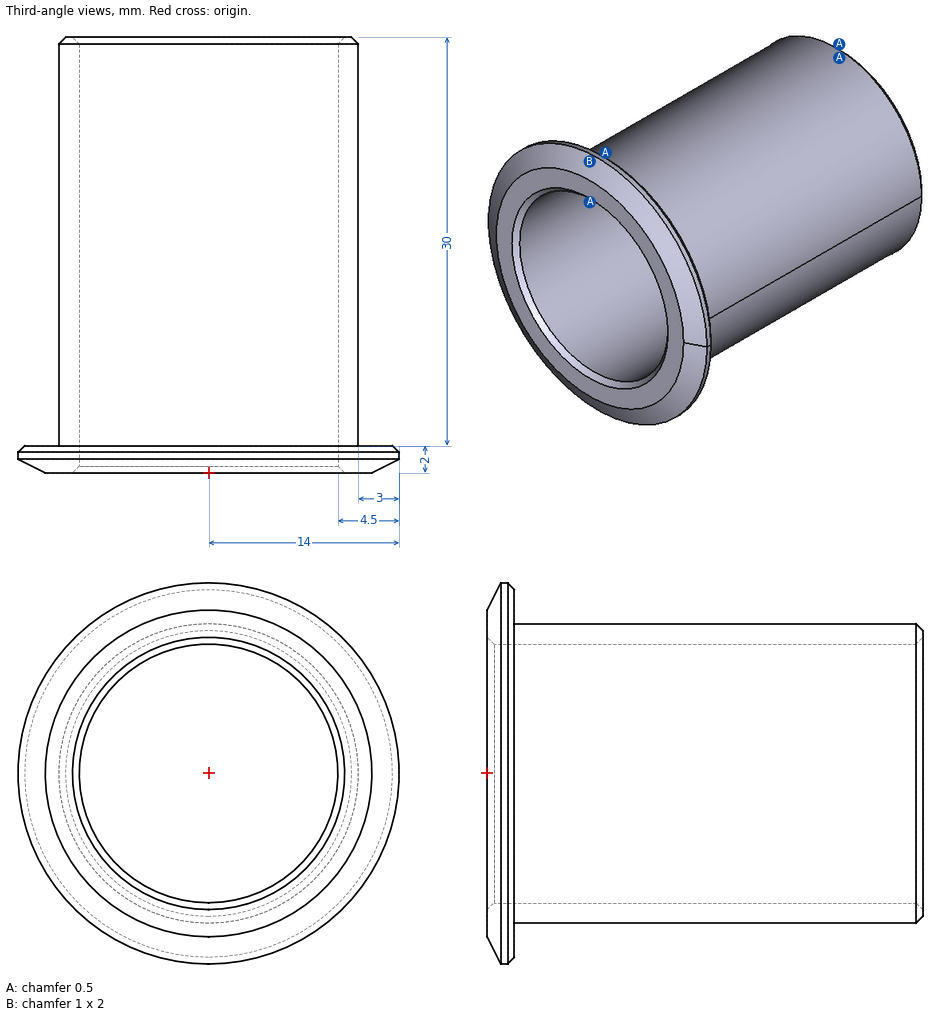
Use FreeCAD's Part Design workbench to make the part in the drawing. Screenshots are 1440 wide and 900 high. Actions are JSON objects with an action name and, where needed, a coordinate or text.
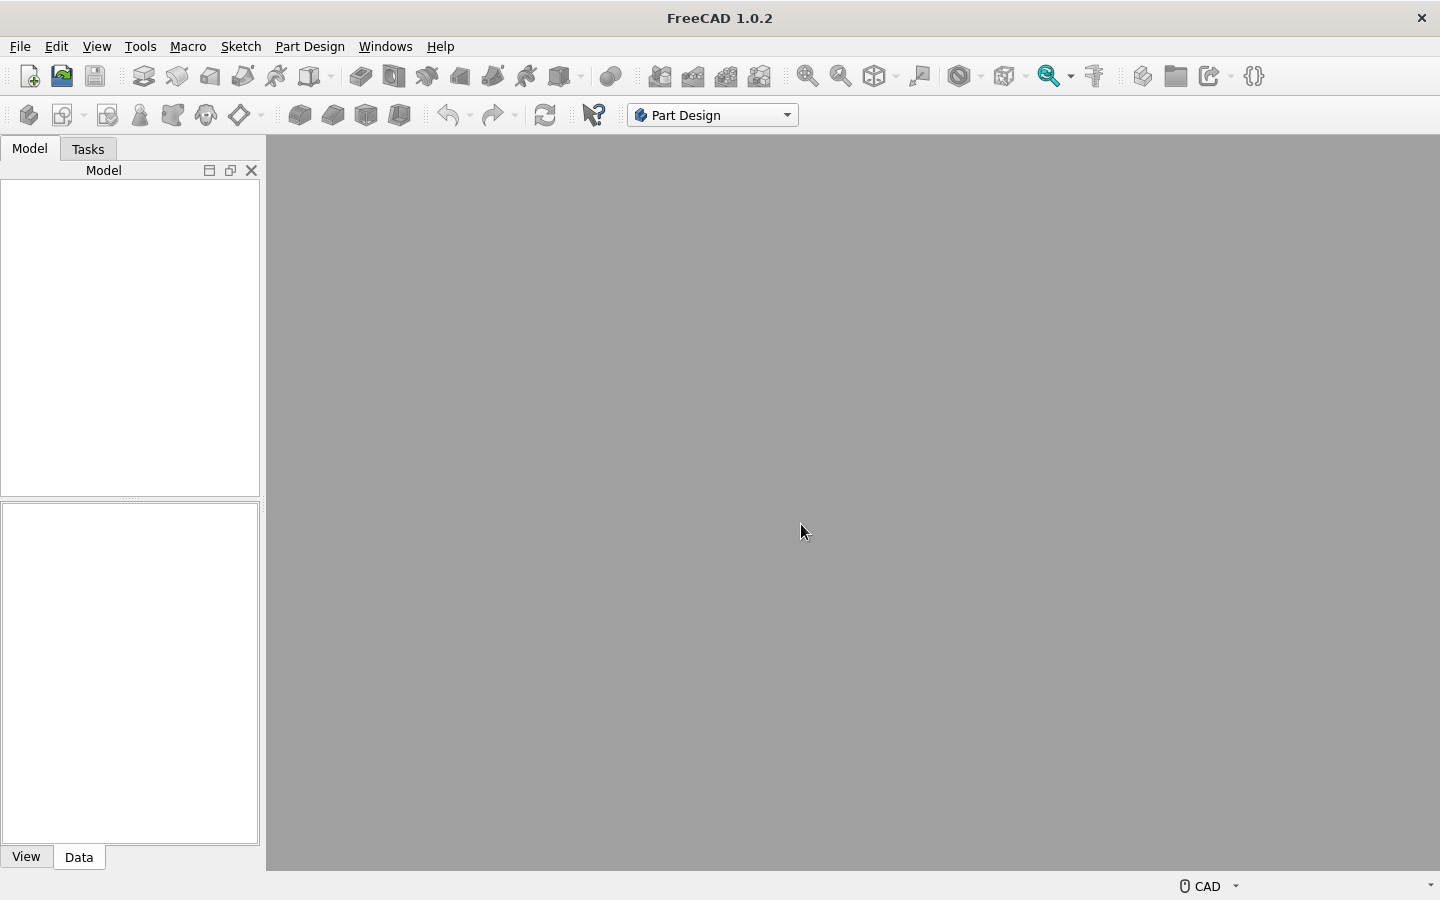
{"action": "key", "text": "ctrl+n"}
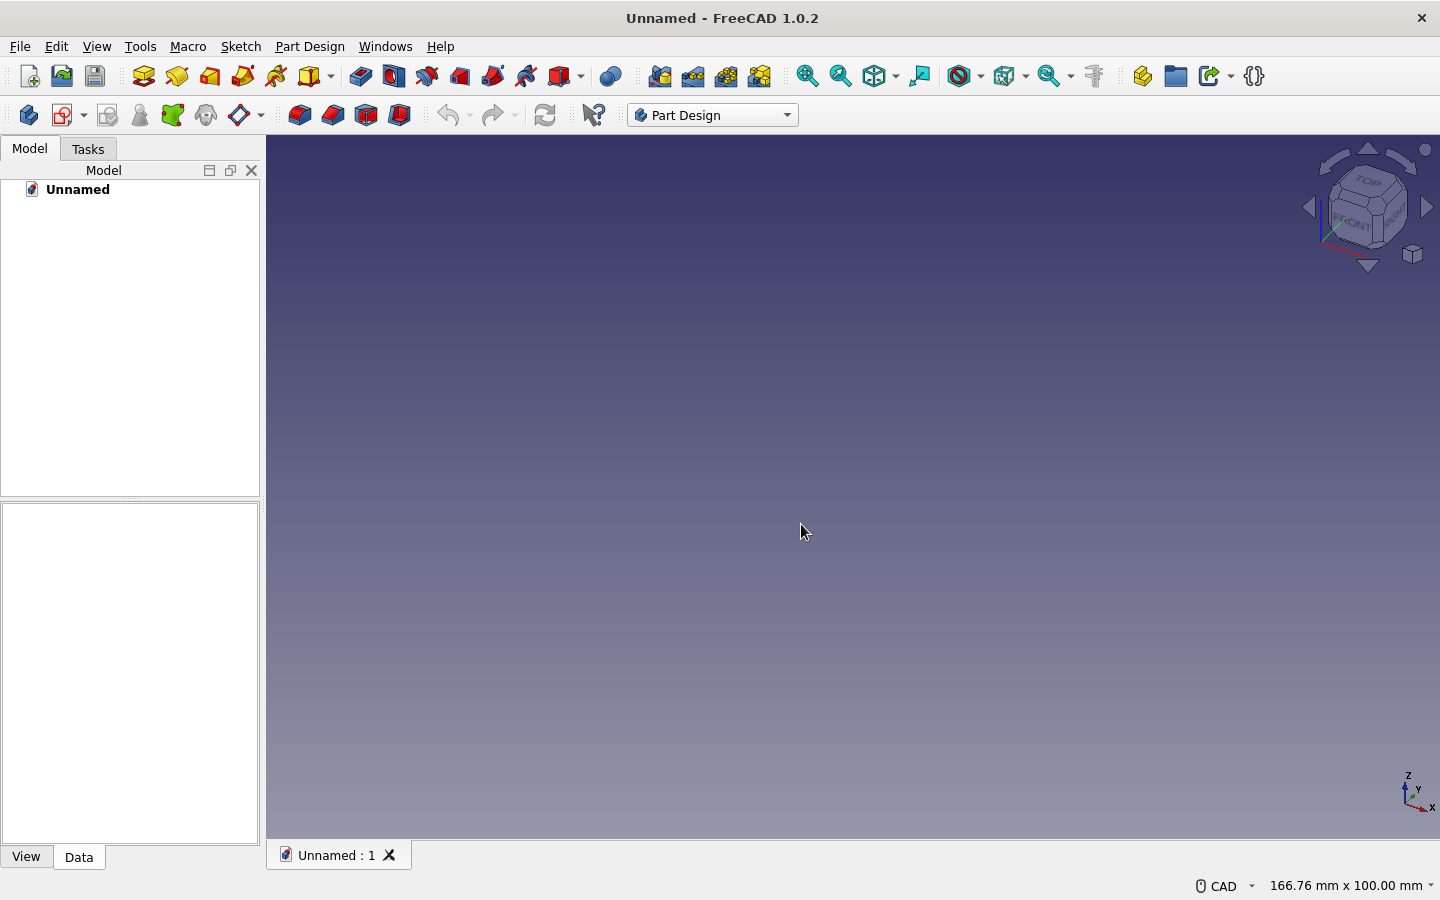
{"action": "left_click", "coordinate": [62, 116]}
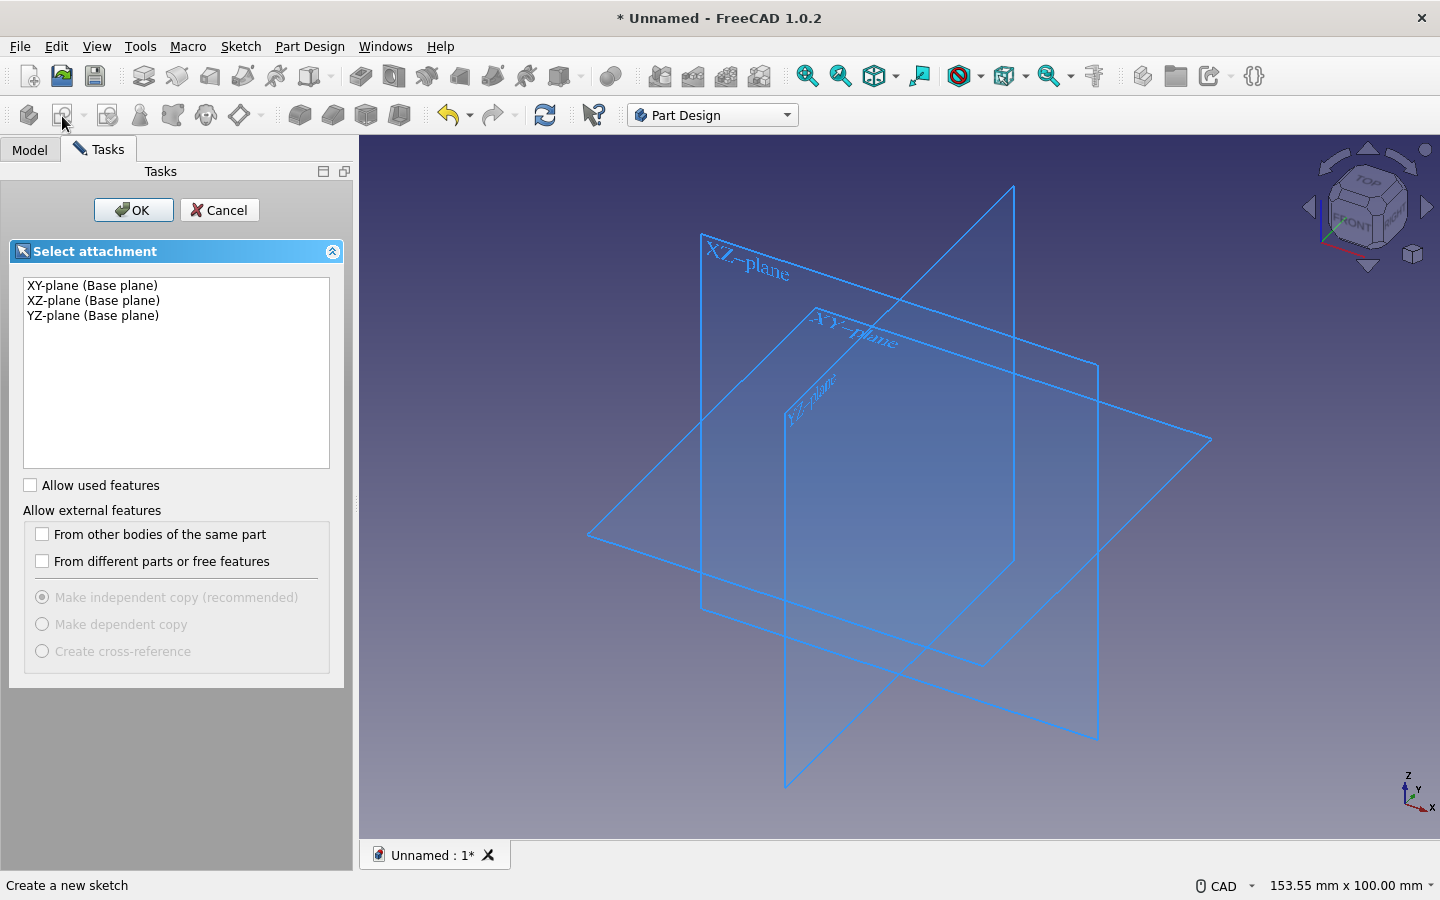
{"action": "left_click", "coordinate": [84, 286]}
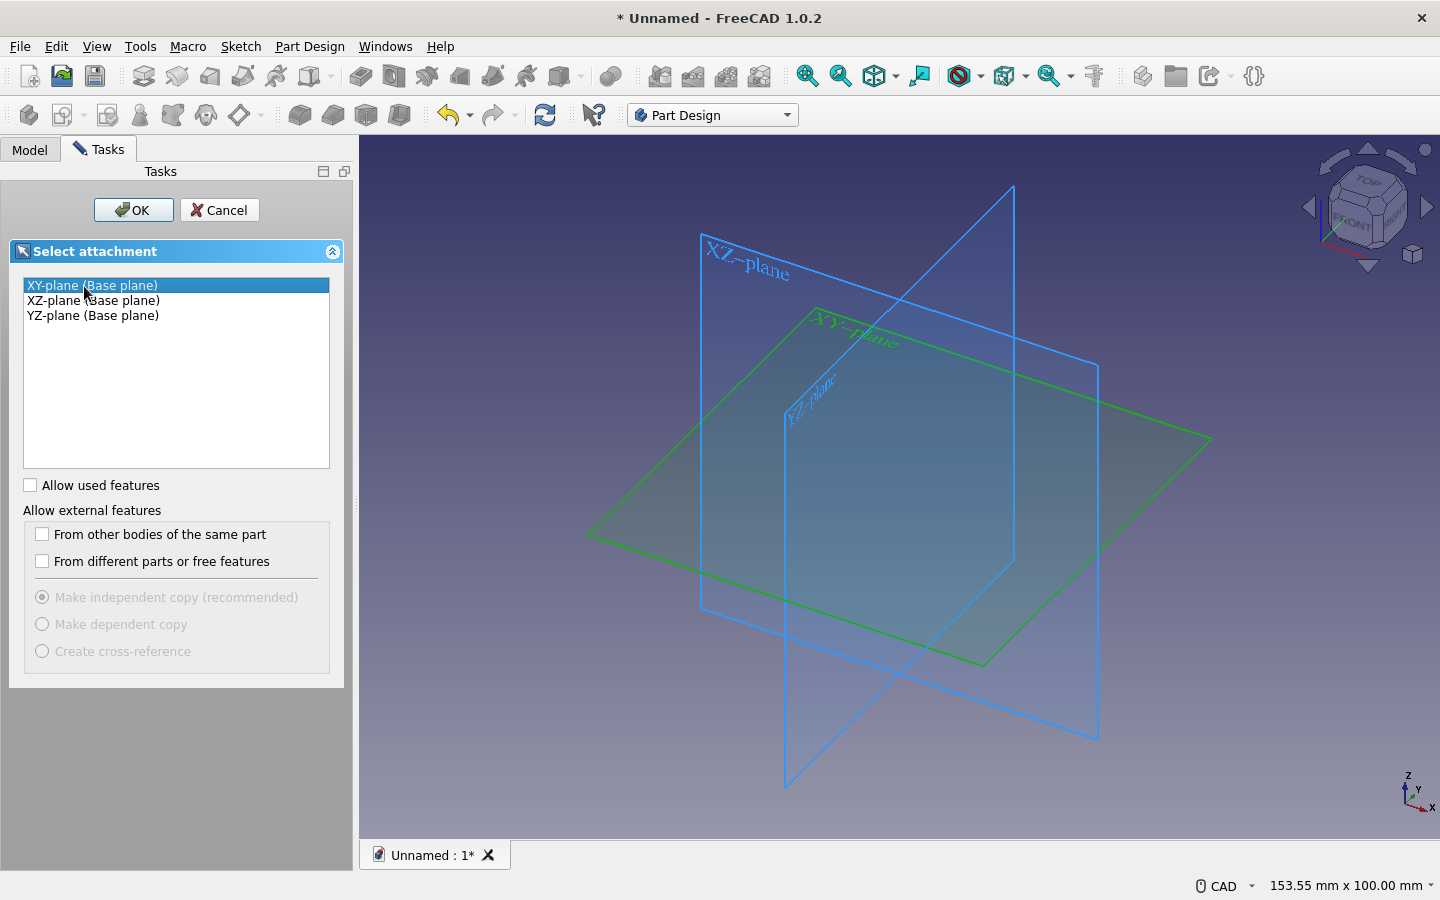
{"action": "left_click", "coordinate": [134, 210]}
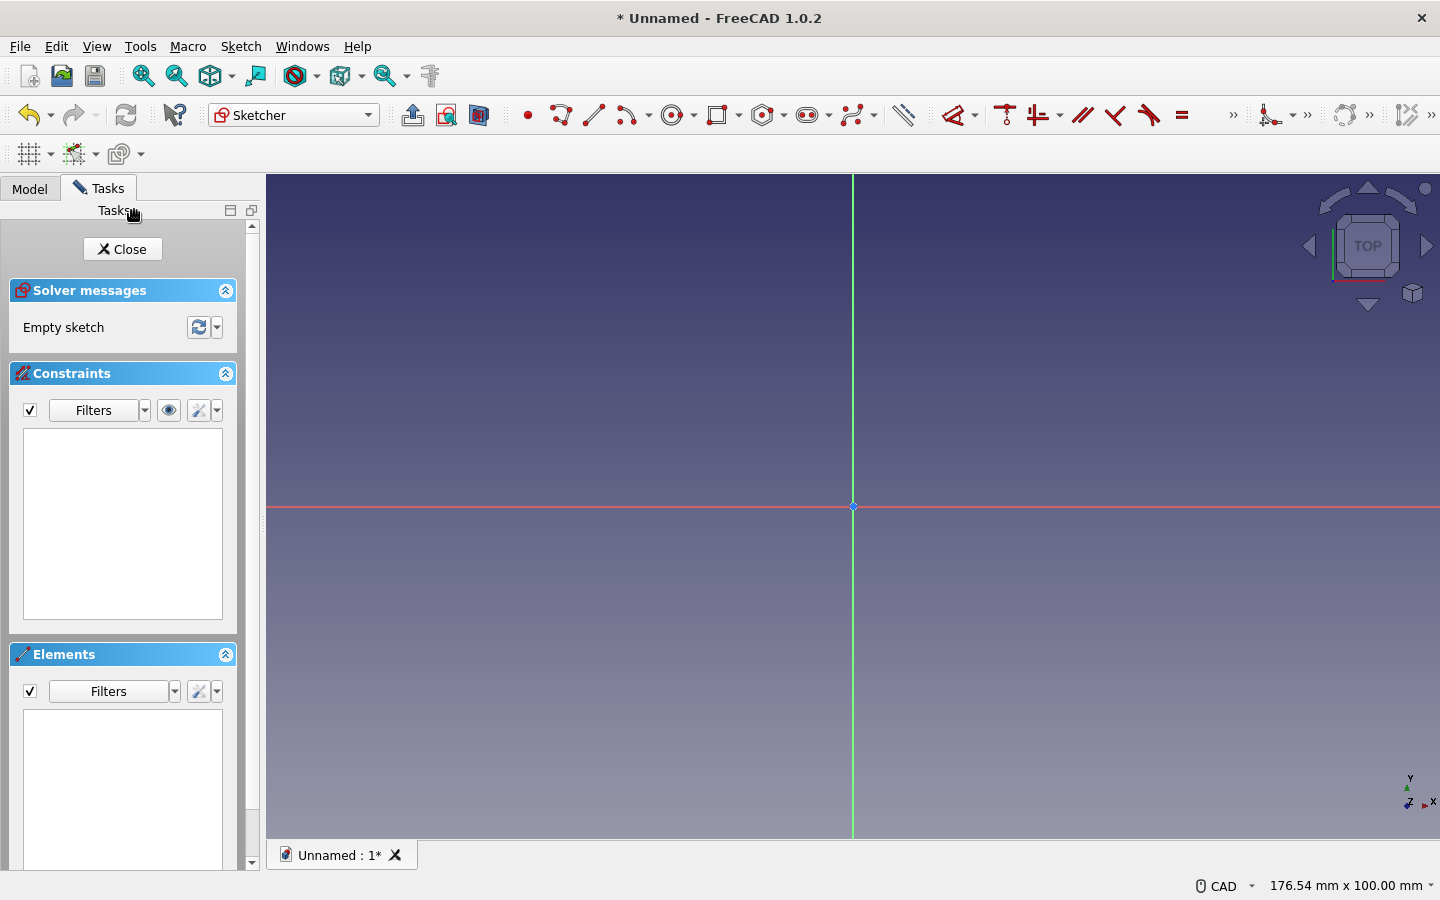
{"action": "scroll", "coordinate": [993, 313], "scroll_direction": "up", "scroll_amount": 4}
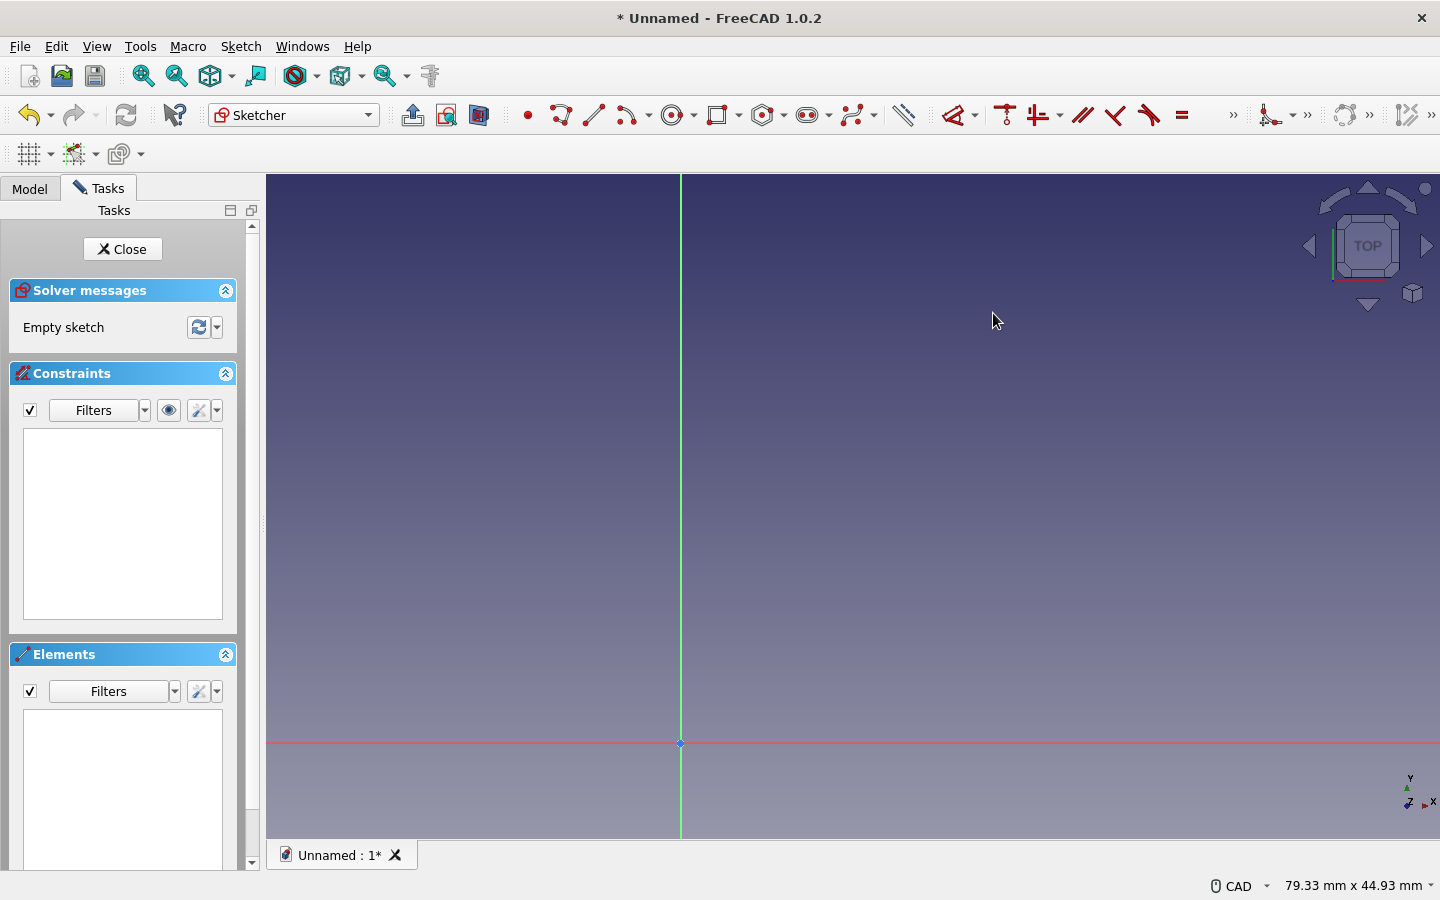
{"action": "left_click", "coordinate": [561, 116]}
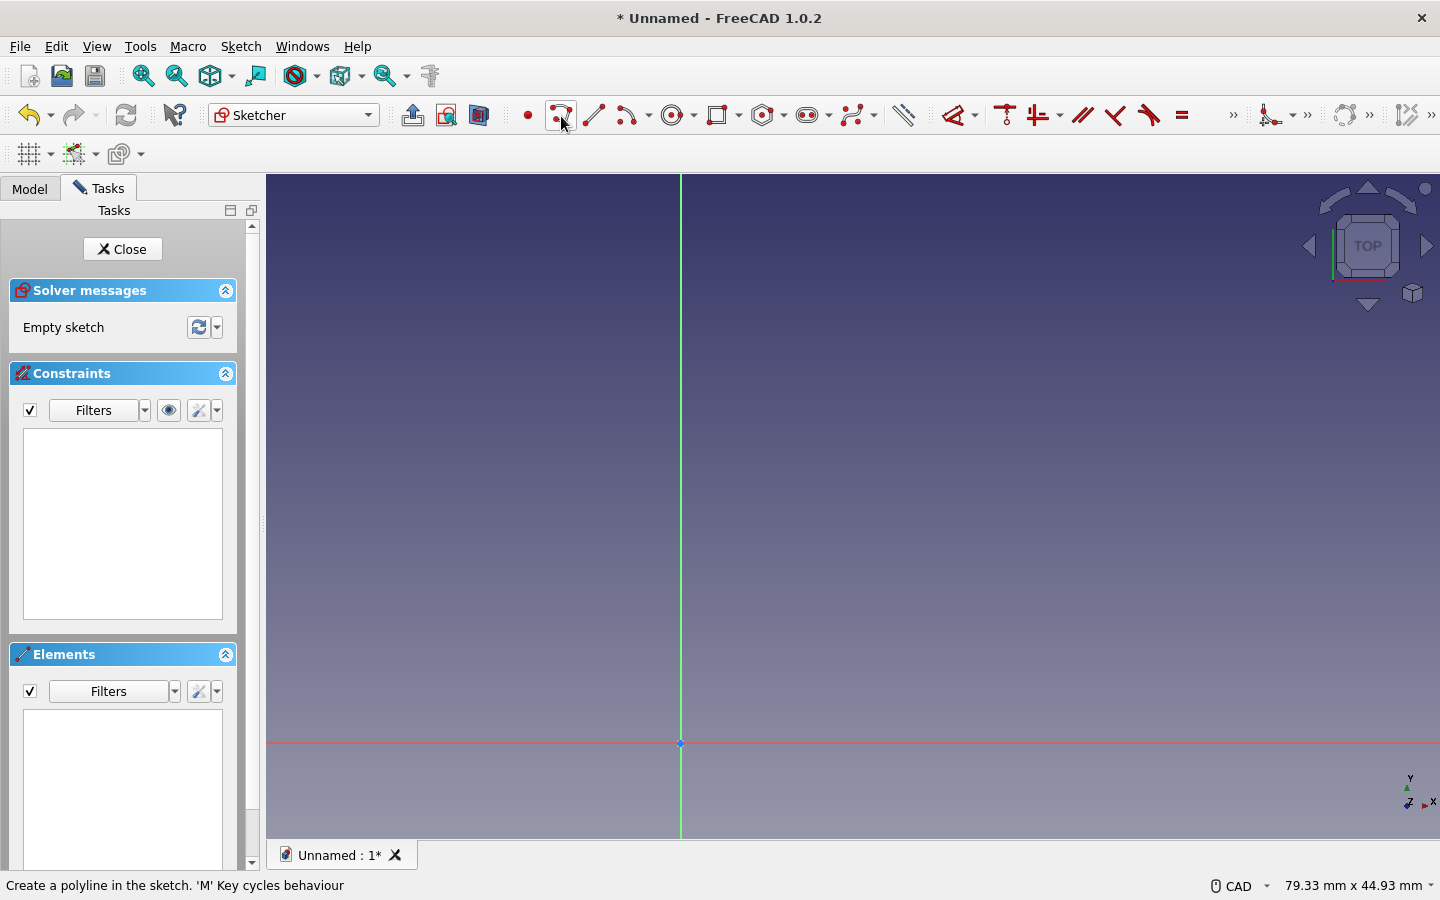
{"action": "left_click", "coordinate": [821, 743]}
{"action": "left_click", "coordinate": [888, 734]}
{"action": "left_click", "coordinate": [888, 714]}
{"action": "left_click", "coordinate": [843, 714]}
{"action": "left_click", "coordinate": [843, 270]}
{"action": "left_click", "coordinate": [821, 270]}
{"action": "left_click", "coordinate": [821, 743]}
{"action": "key", "text": "Escape"}
{"action": "key", "text": "Escape"}